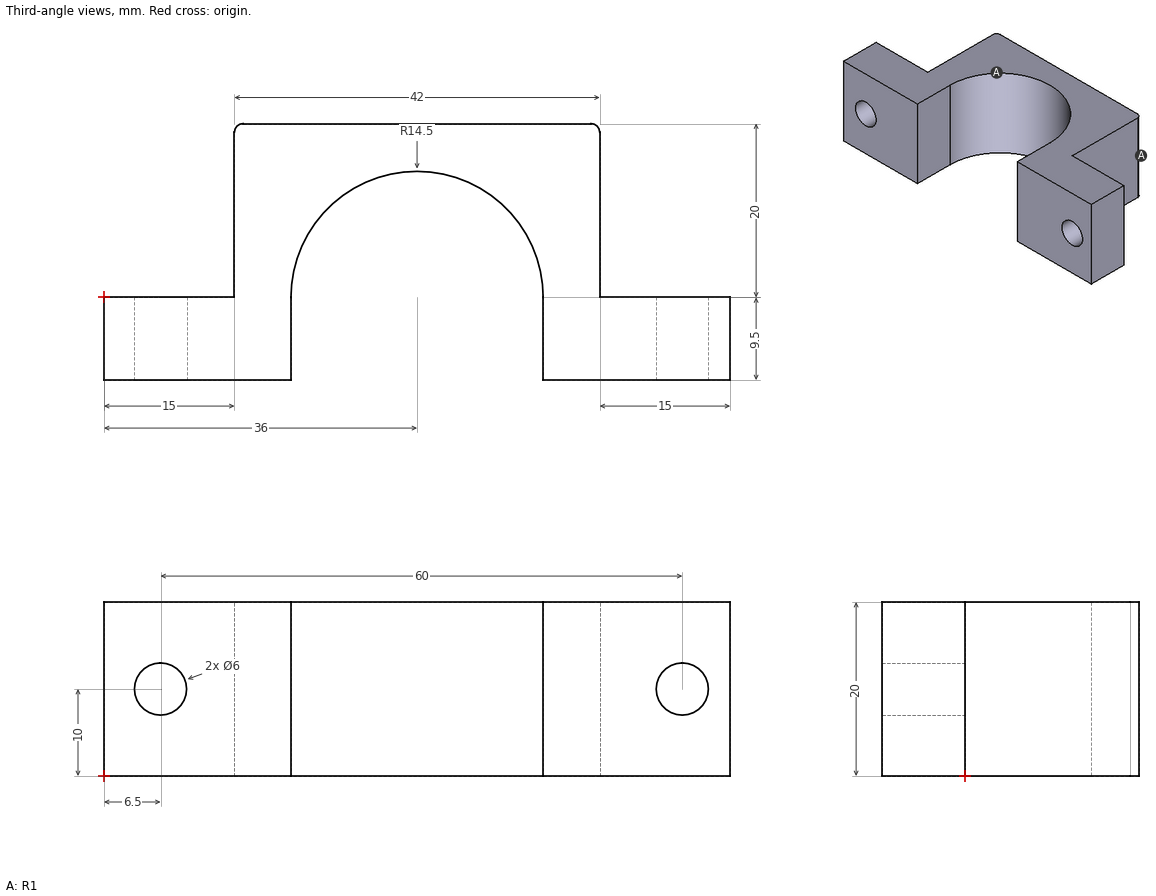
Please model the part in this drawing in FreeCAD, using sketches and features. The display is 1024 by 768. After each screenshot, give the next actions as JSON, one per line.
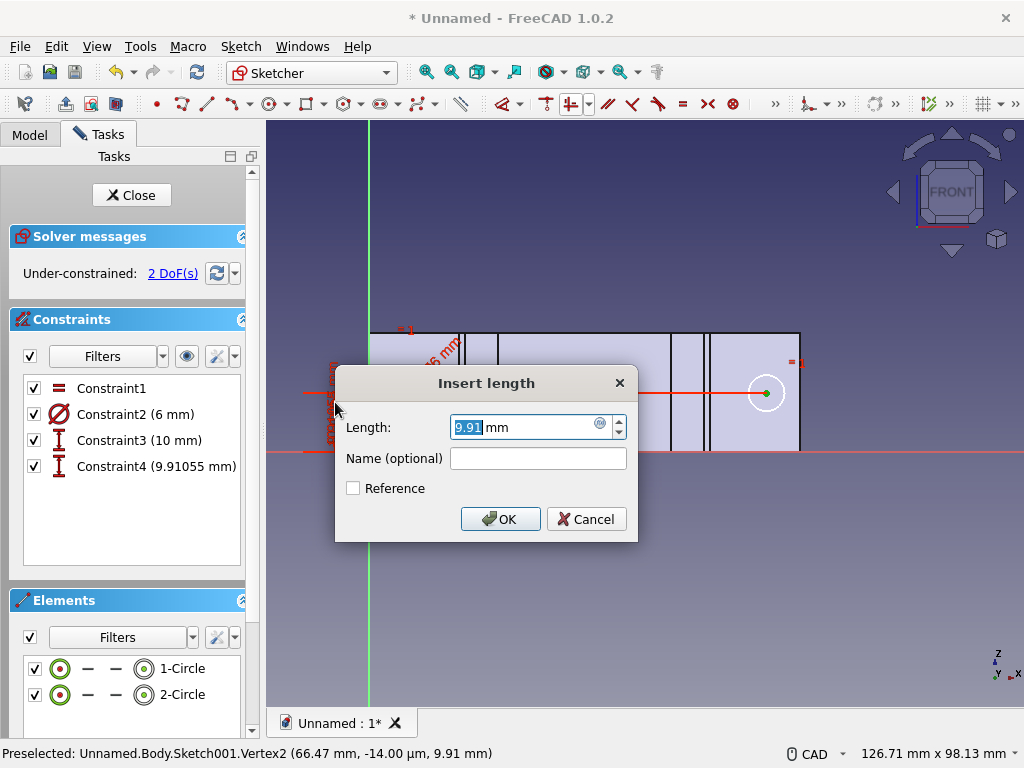
{"action": "type", "text": "10"}
{"action": "key", "text": "Return"}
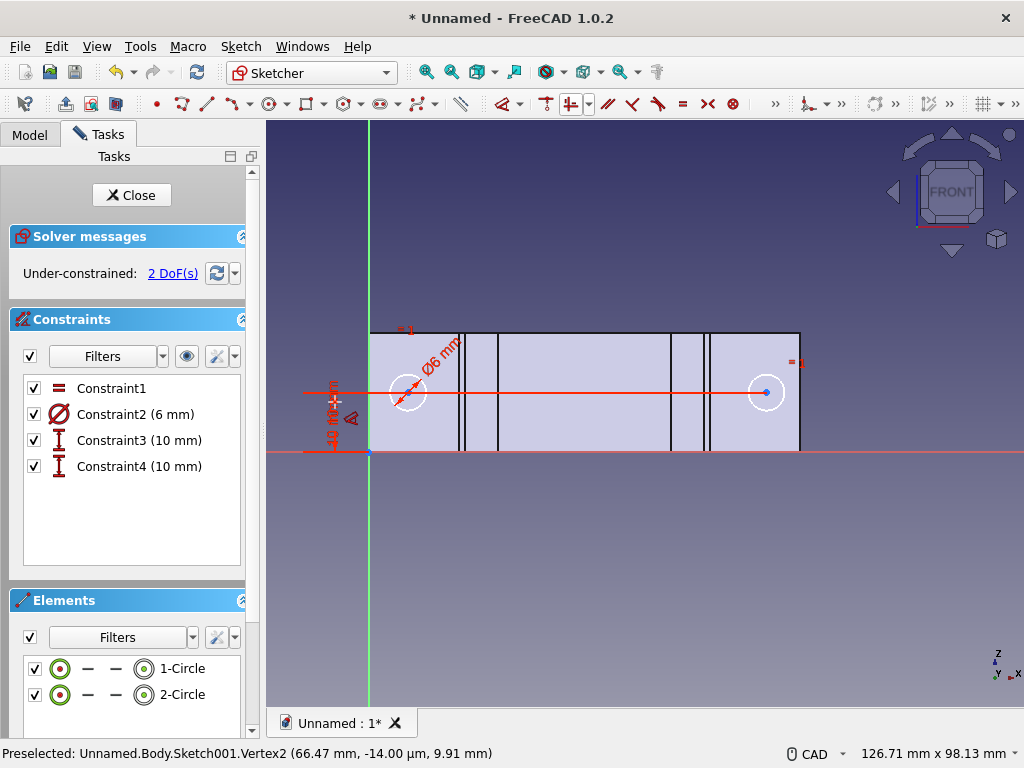
{"action": "left_click", "coordinate": [408, 393]}
{"action": "left_click", "coordinate": [388, 486]}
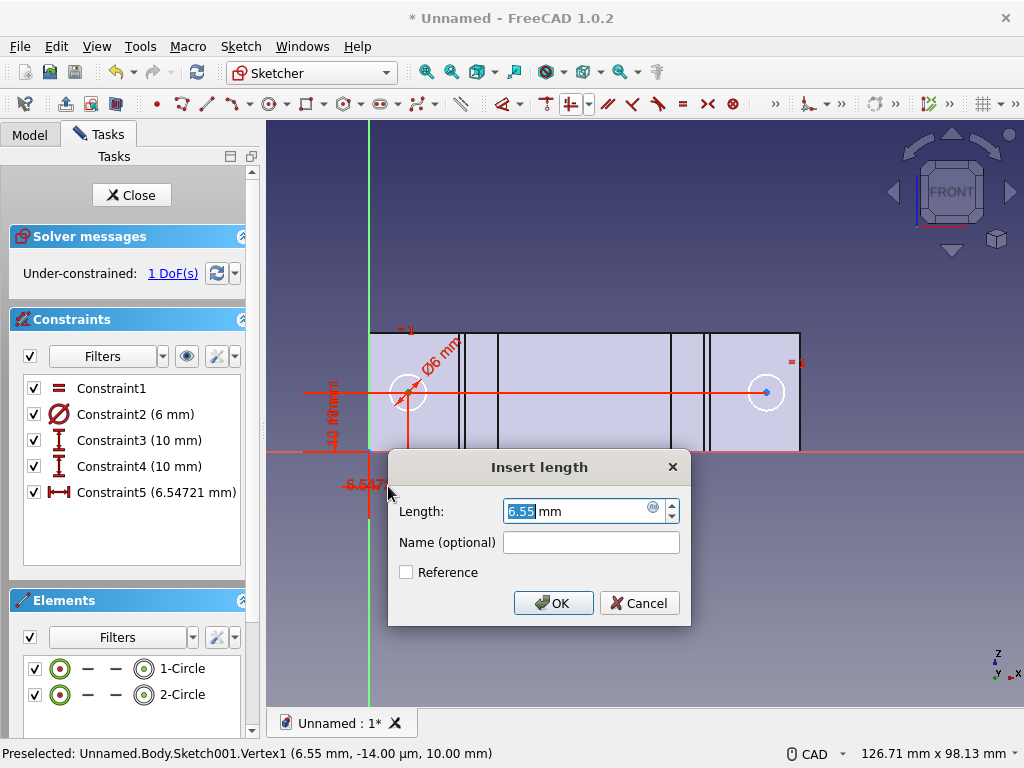
{"action": "type", "text": "6.5"}
{"action": "key", "text": "Return"}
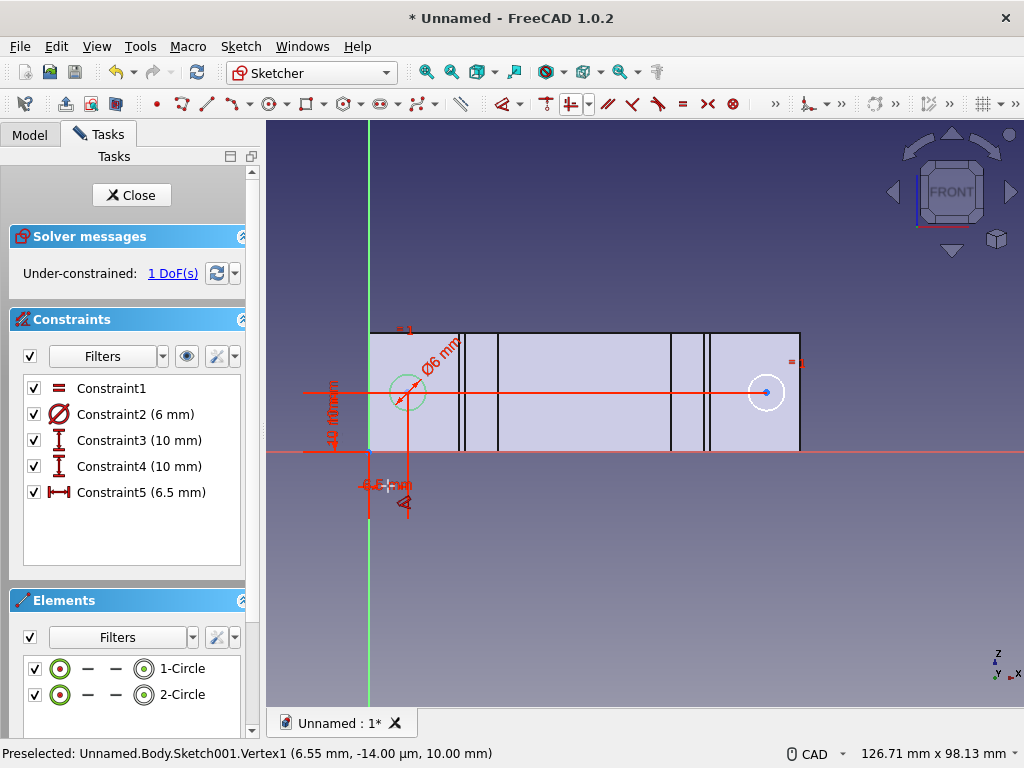
{"action": "left_click", "coordinate": [408, 393]}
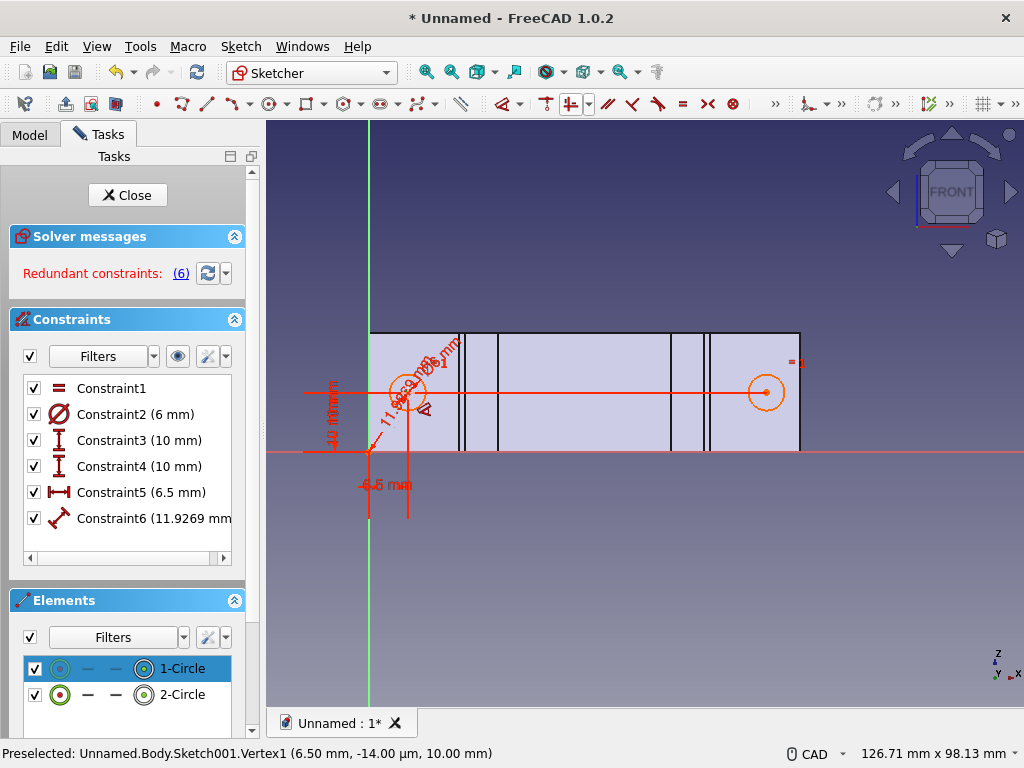
{"action": "left_click", "coordinate": [767, 393]}
{"action": "left_click", "coordinate": [587, 359]}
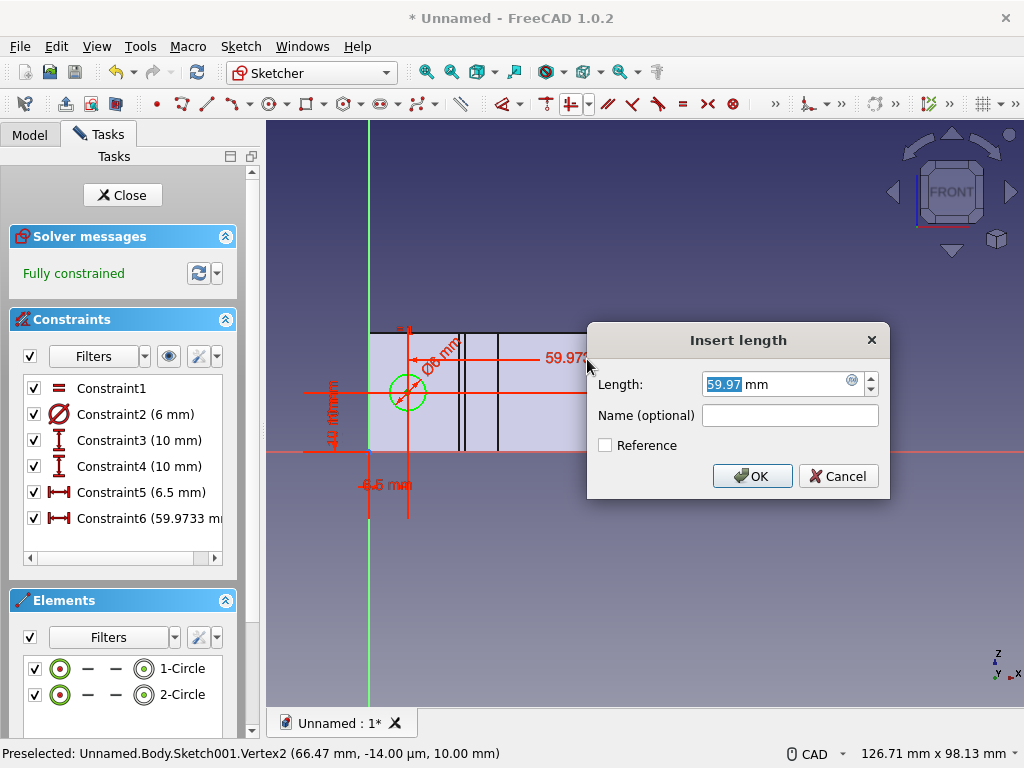
{"action": "type", "text": "60"}
{"action": "key", "text": "Return"}
{"action": "key", "text": "Escape"}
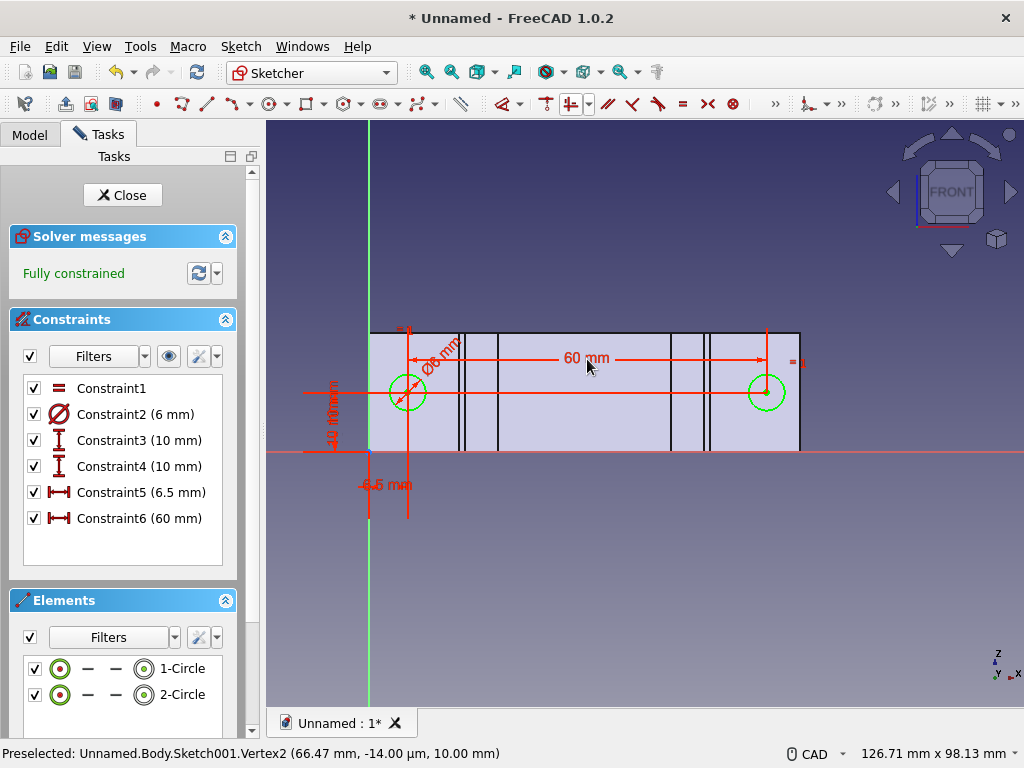
{"action": "left_click", "coordinate": [123, 195]}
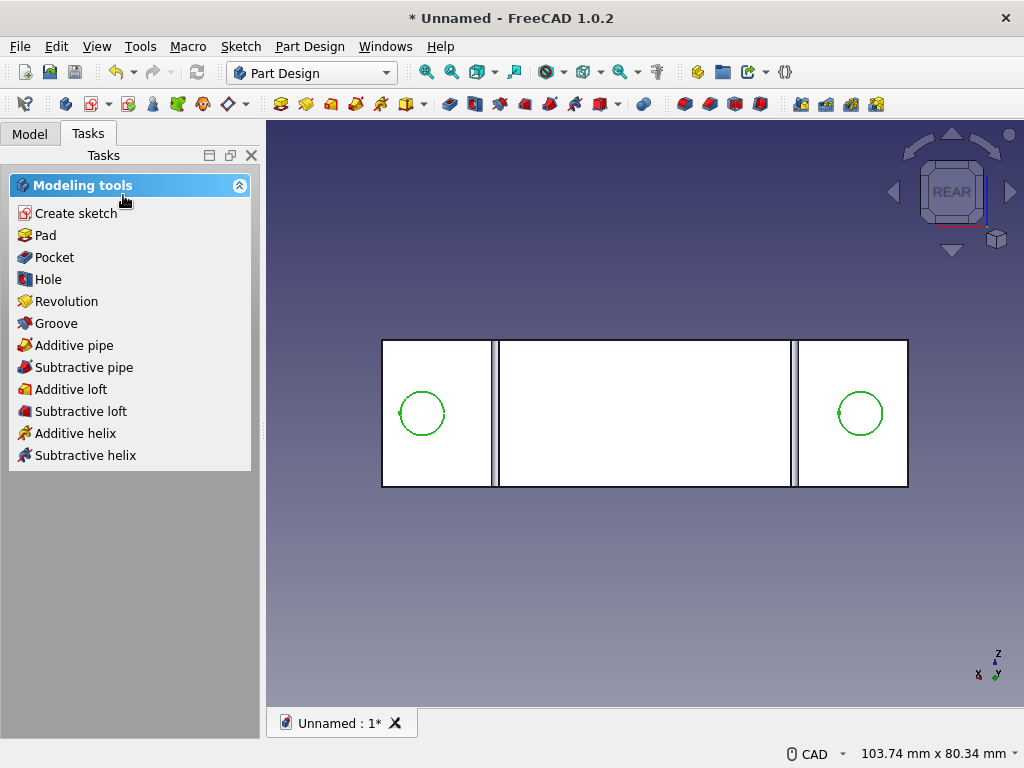
{"action": "left_click", "coordinate": [450, 104]}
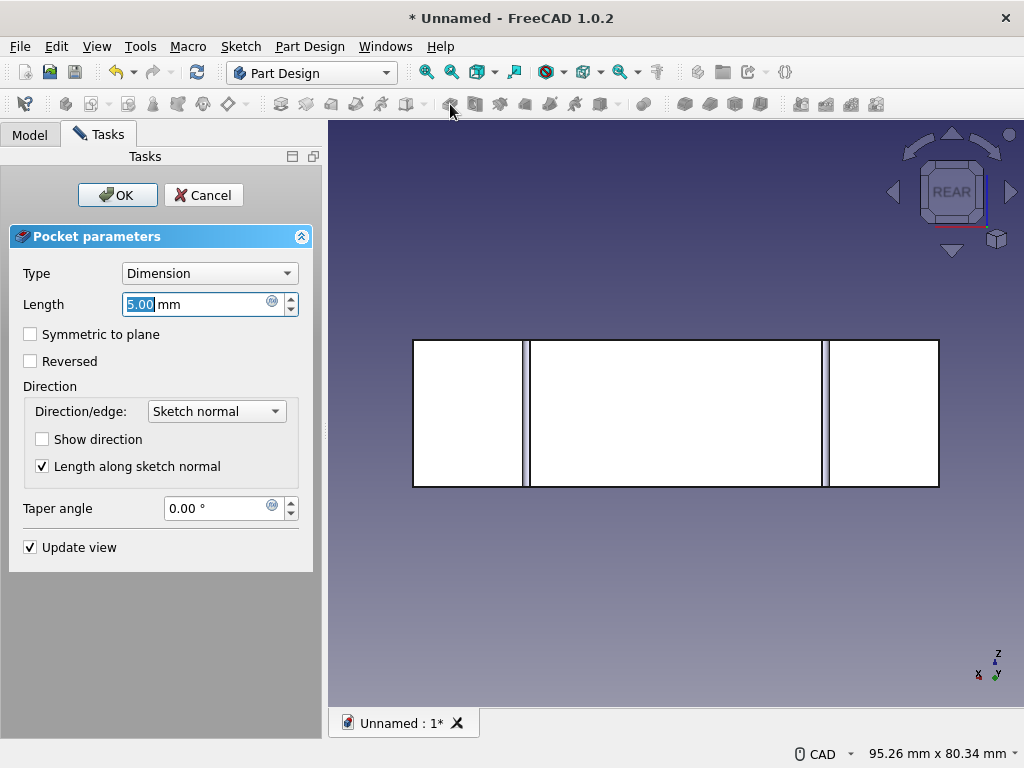
{"action": "left_click", "coordinate": [210, 274]}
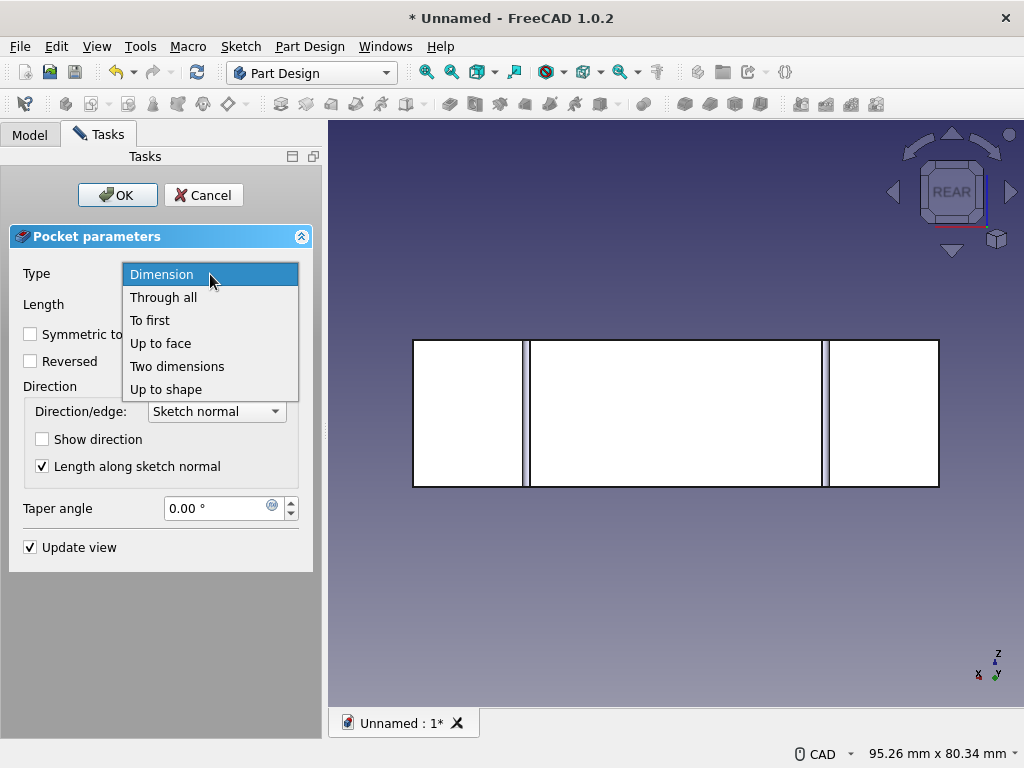
{"action": "left_click", "coordinate": [208, 298]}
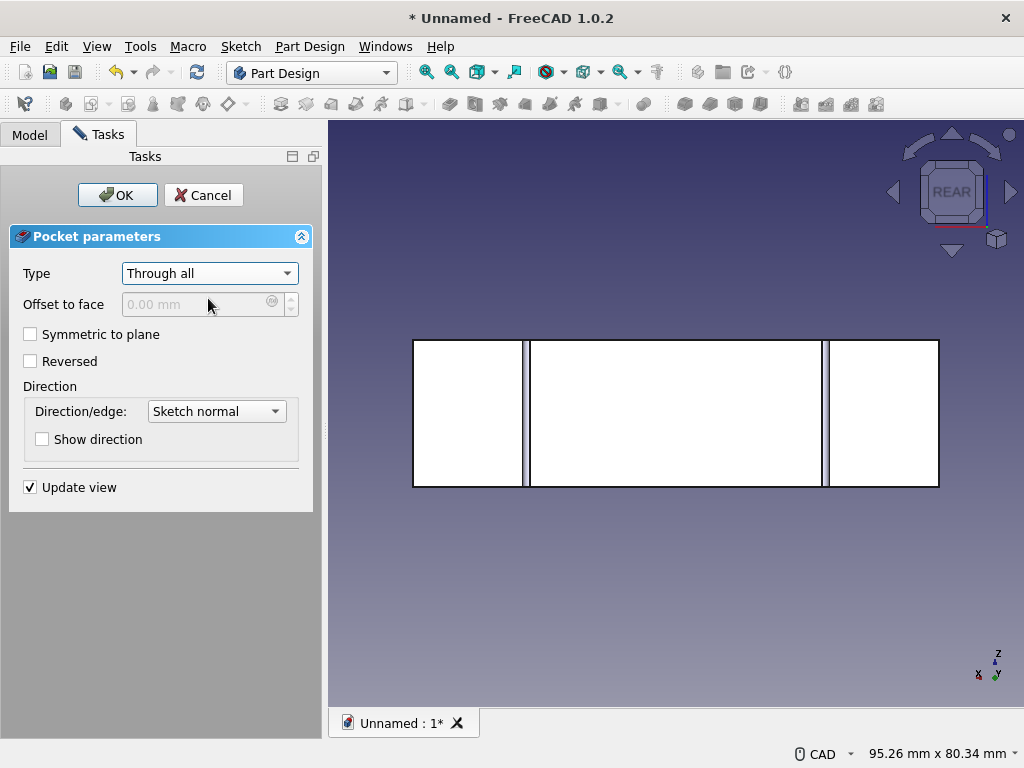
{"action": "left_click", "coordinate": [31, 361]}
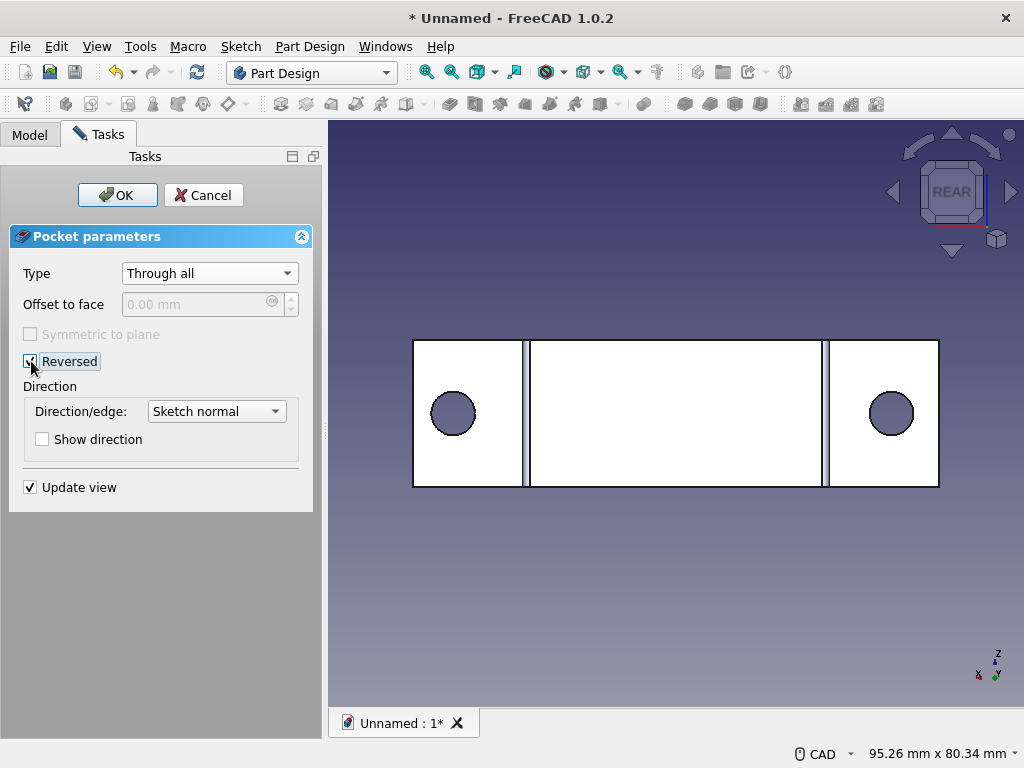
{"action": "left_click", "coordinate": [118, 195]}